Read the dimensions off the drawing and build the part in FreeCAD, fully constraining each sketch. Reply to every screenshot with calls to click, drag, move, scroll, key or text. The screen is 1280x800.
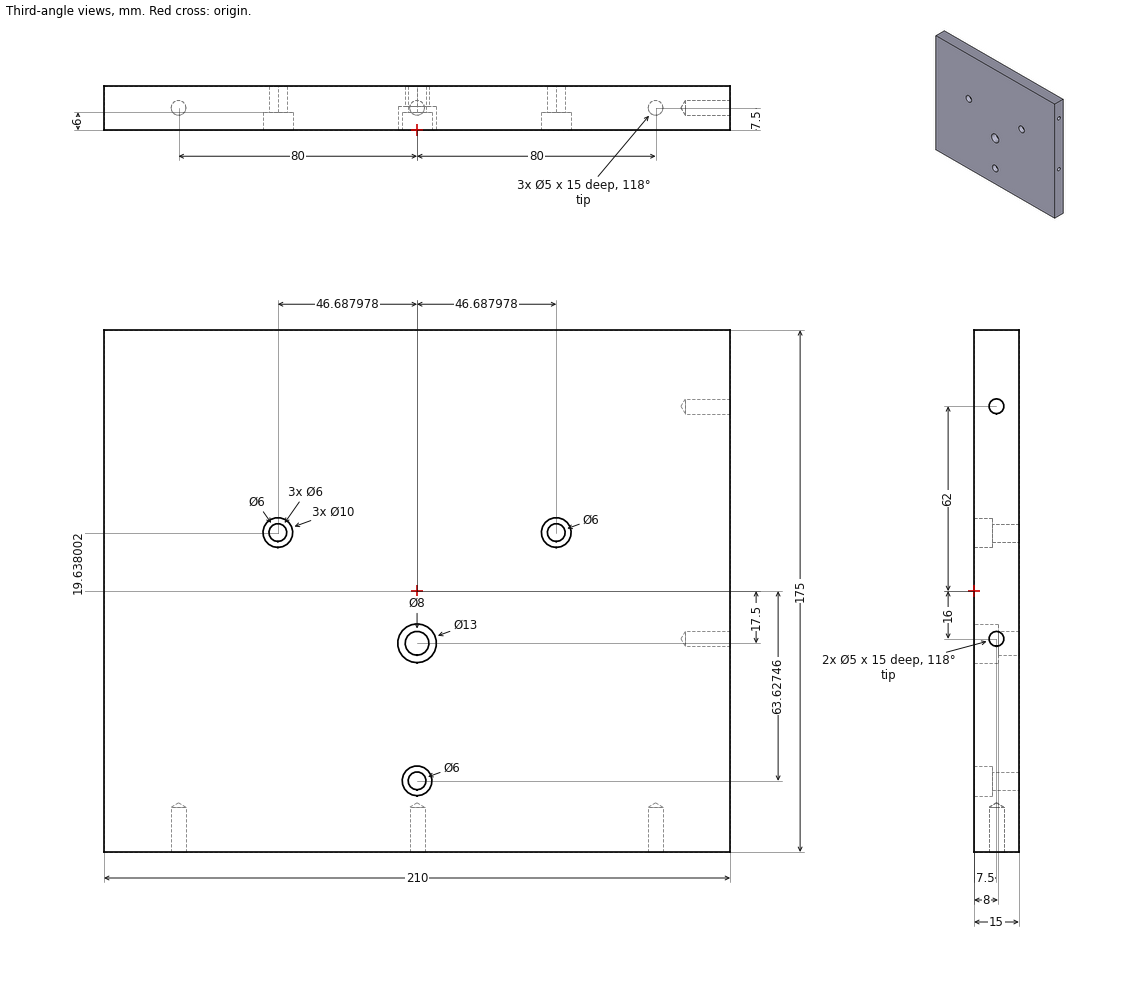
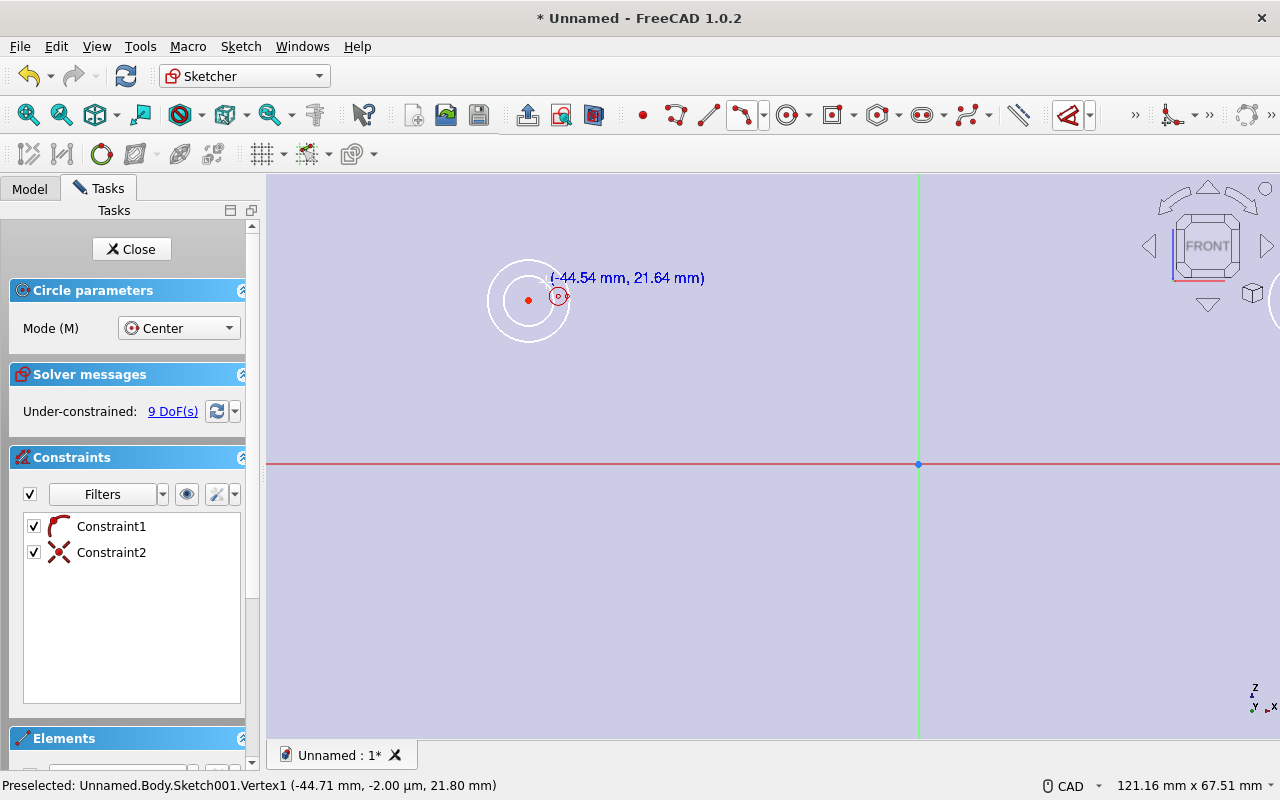
scroll(530, 300, down, 4)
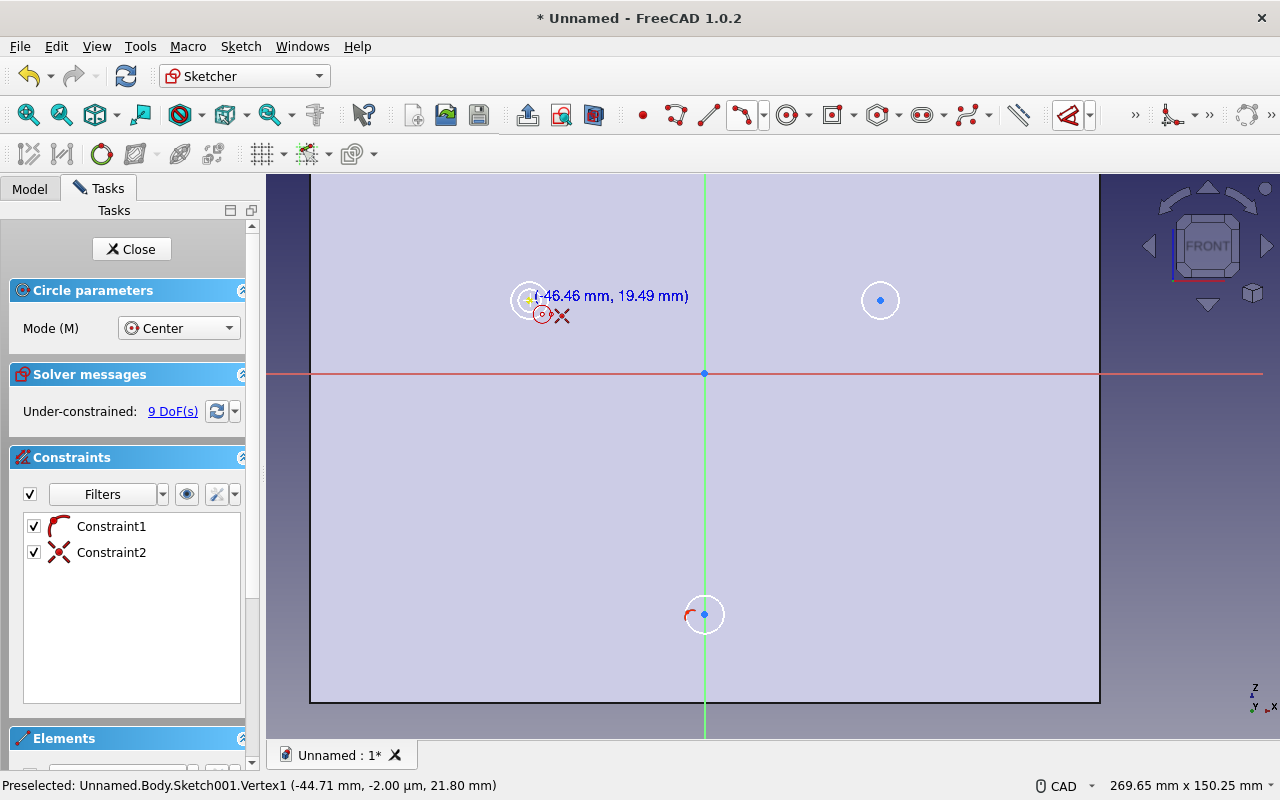
scroll(880, 300, up, 4)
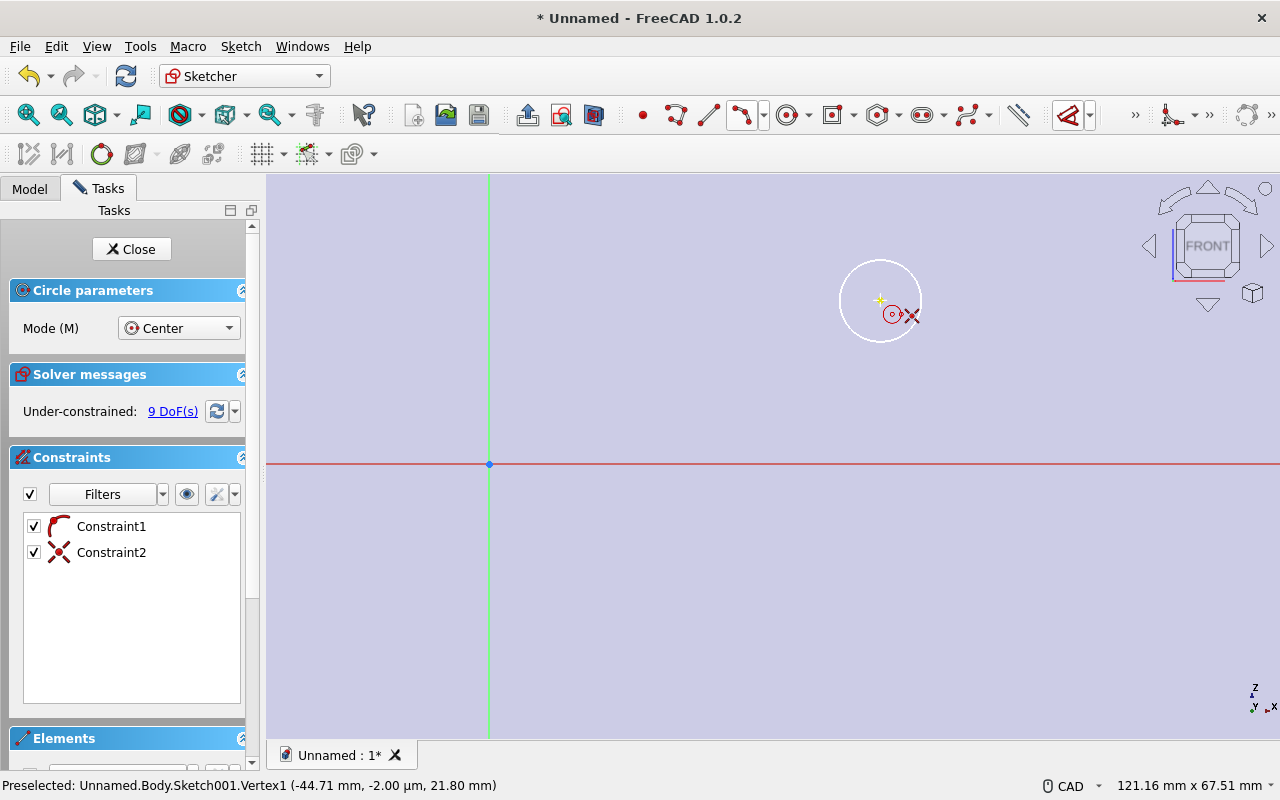
click(880, 301)
click(898, 282)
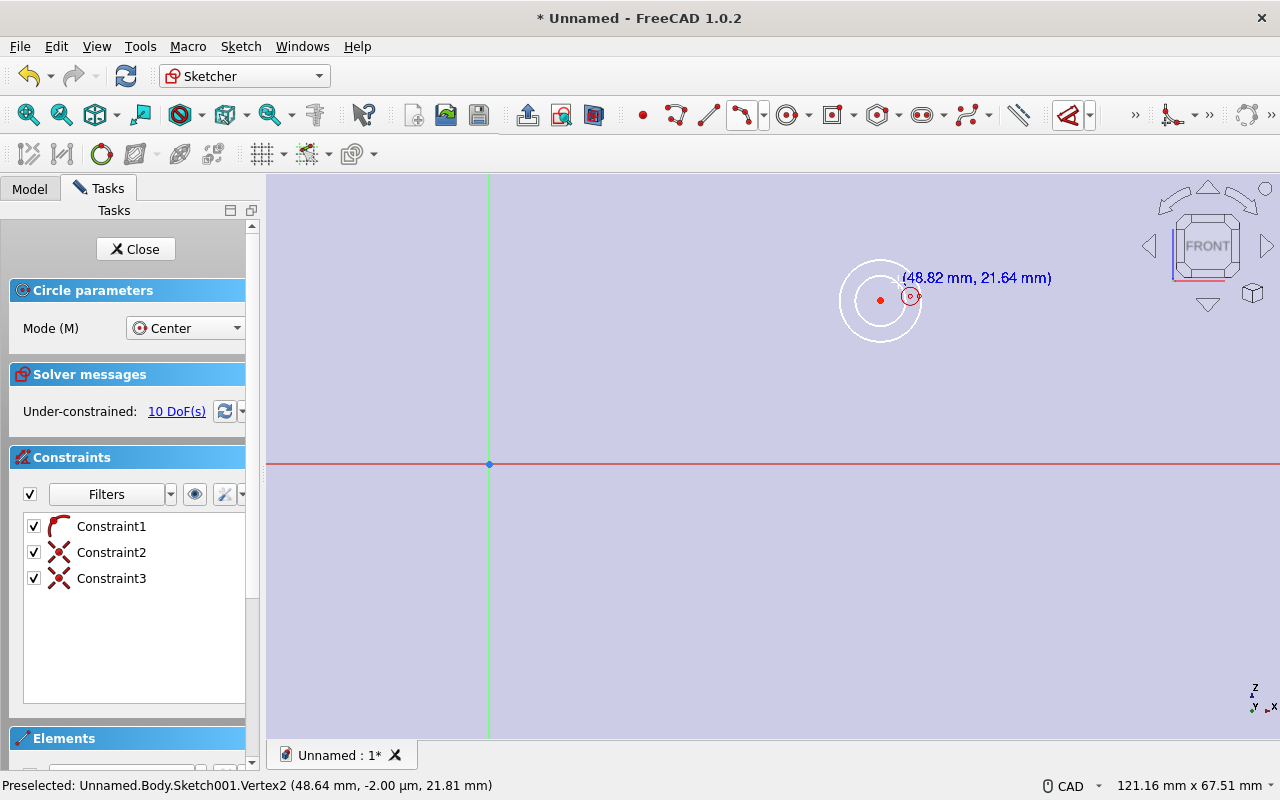
scroll(880, 300, down, 4)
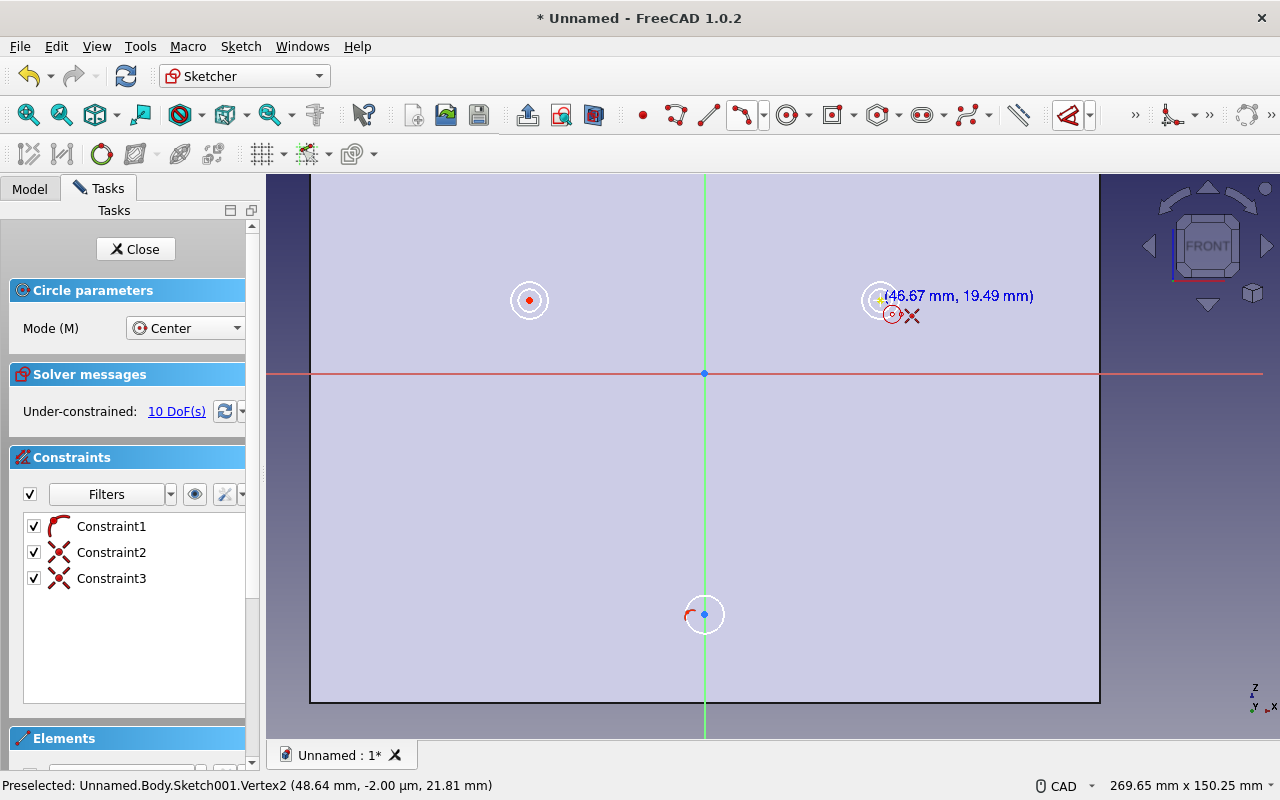
scroll(705, 613, up, 4)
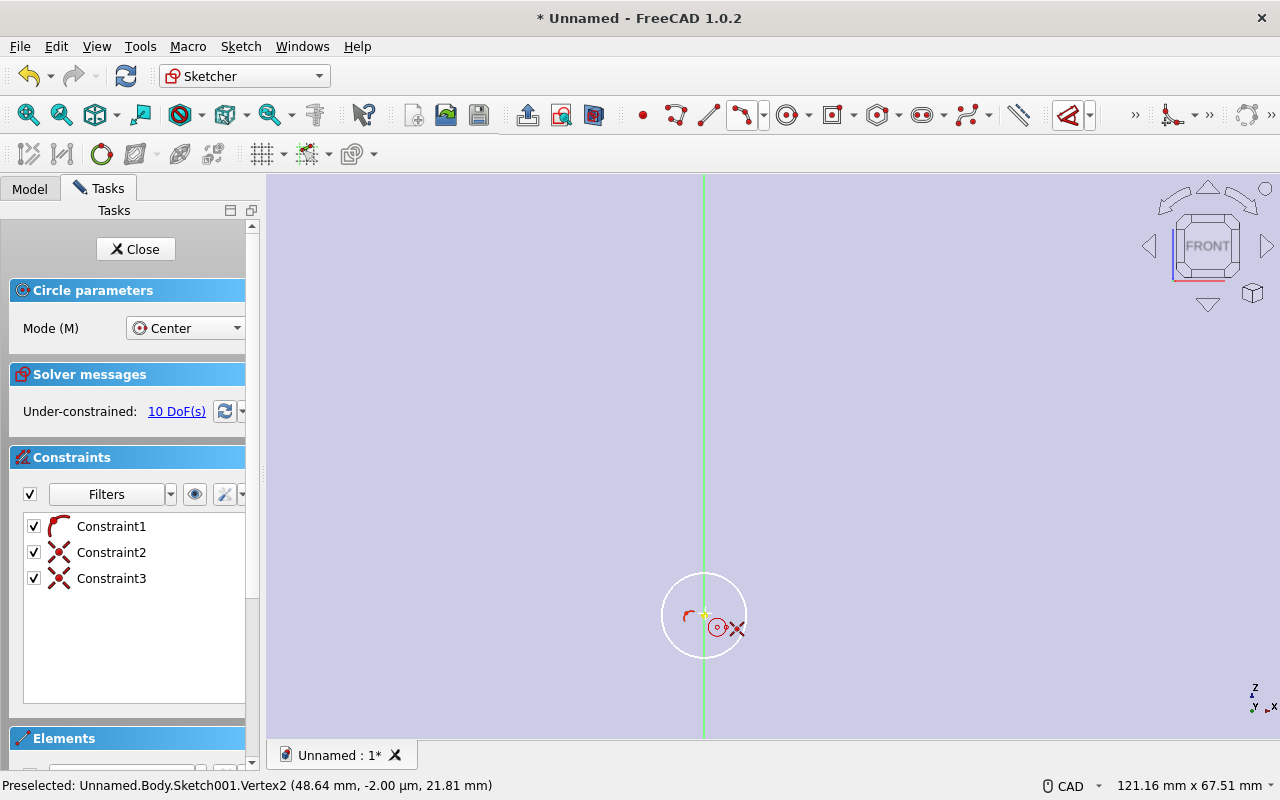
click(704, 615)
click(722, 595)
key(Escape)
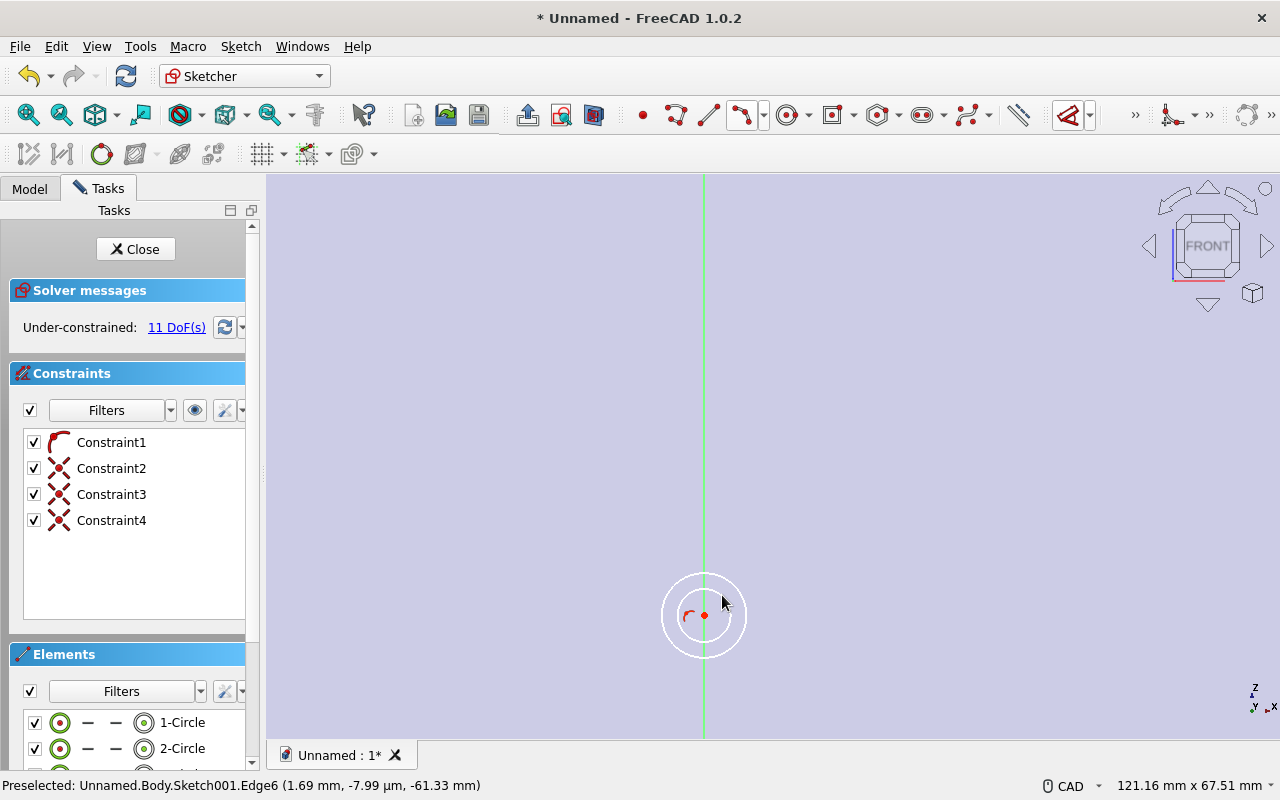
scroll(705, 614, down, 4)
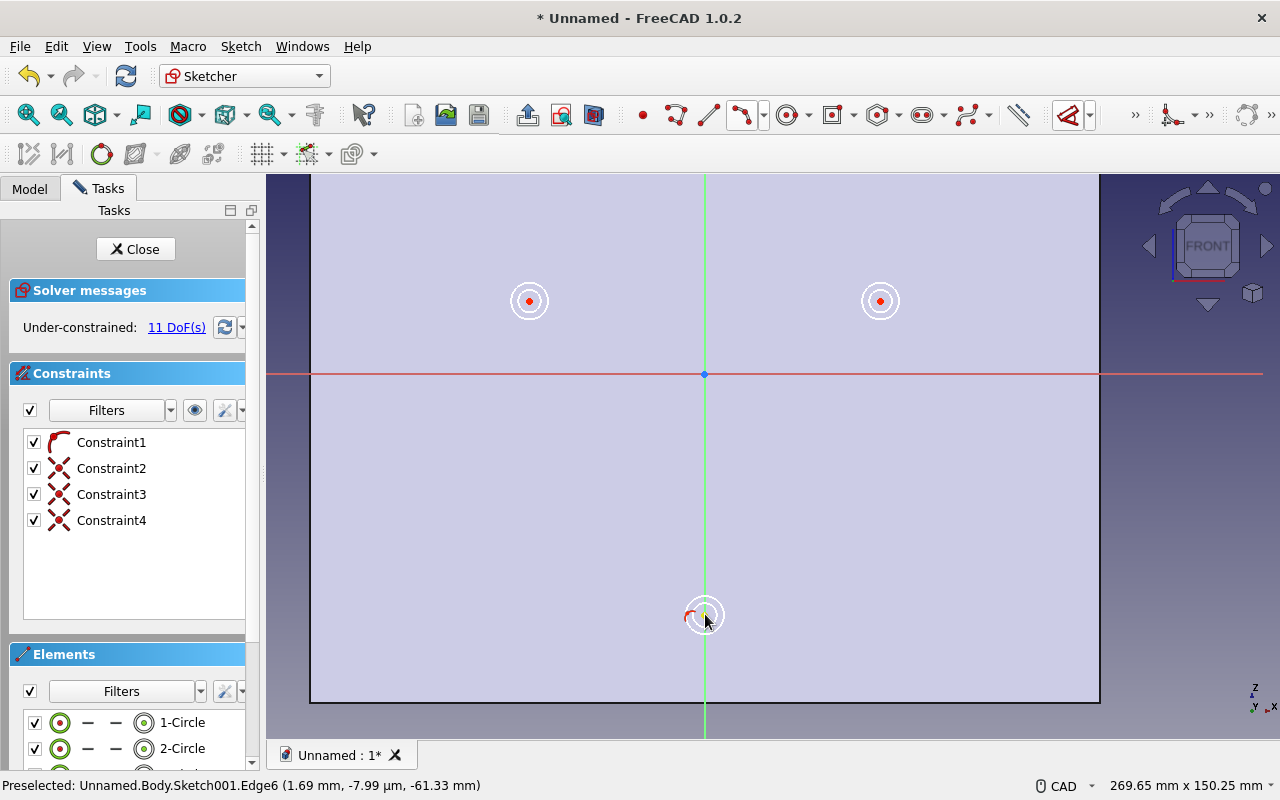
scroll(543, 288, up, 4)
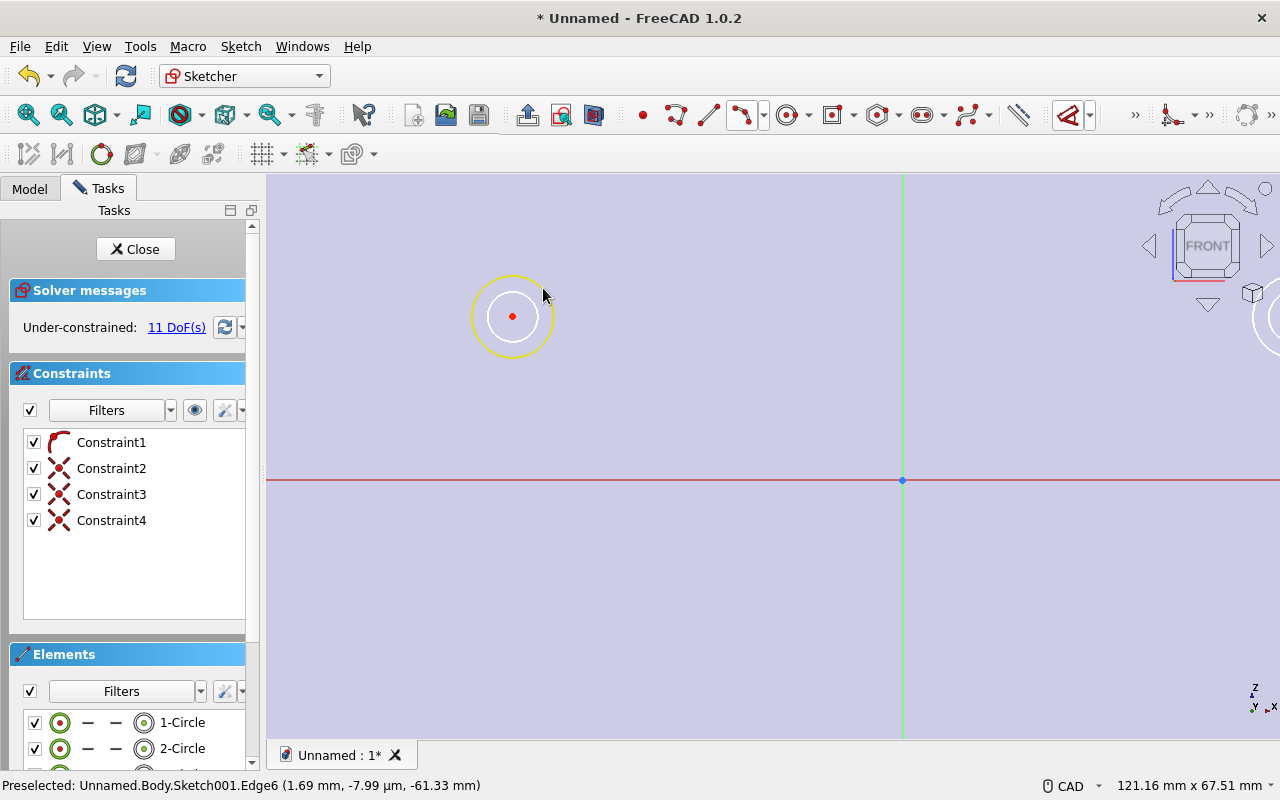
click(542, 288)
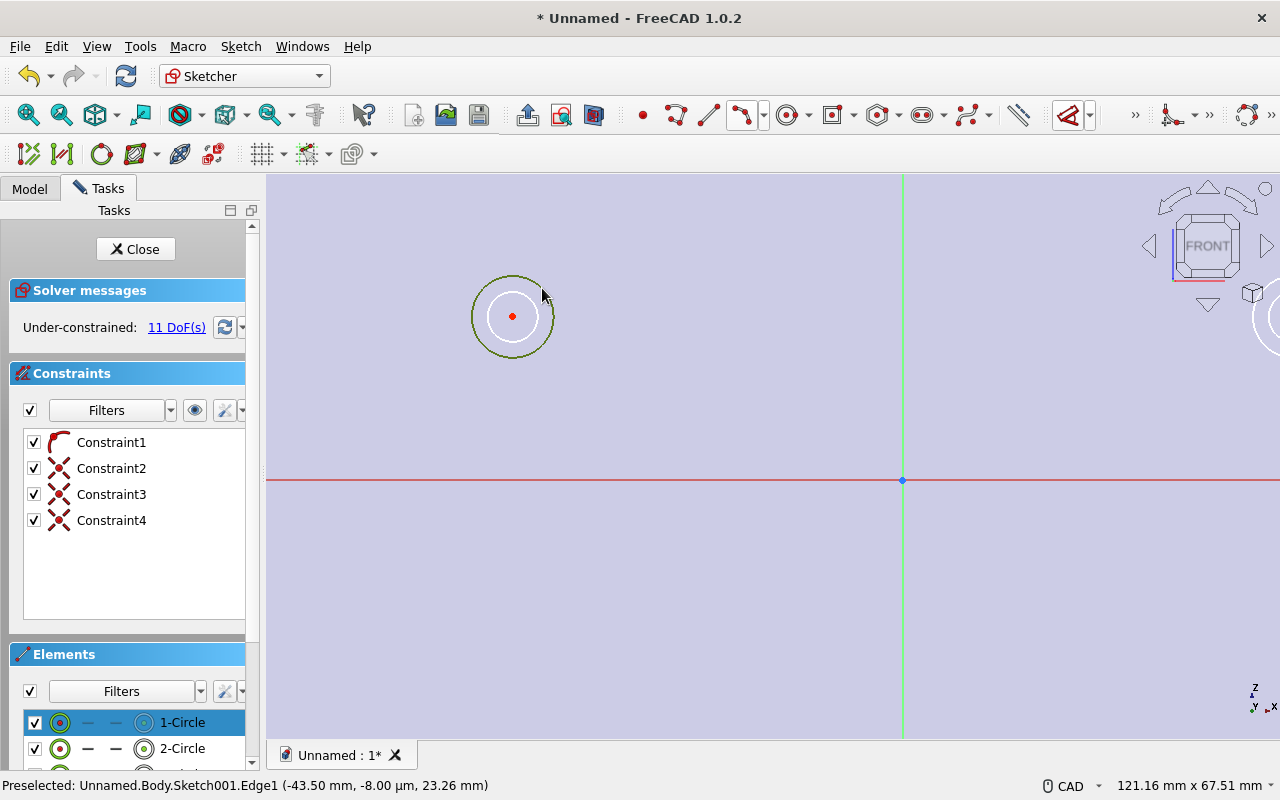
scroll(543, 287, down, 4)